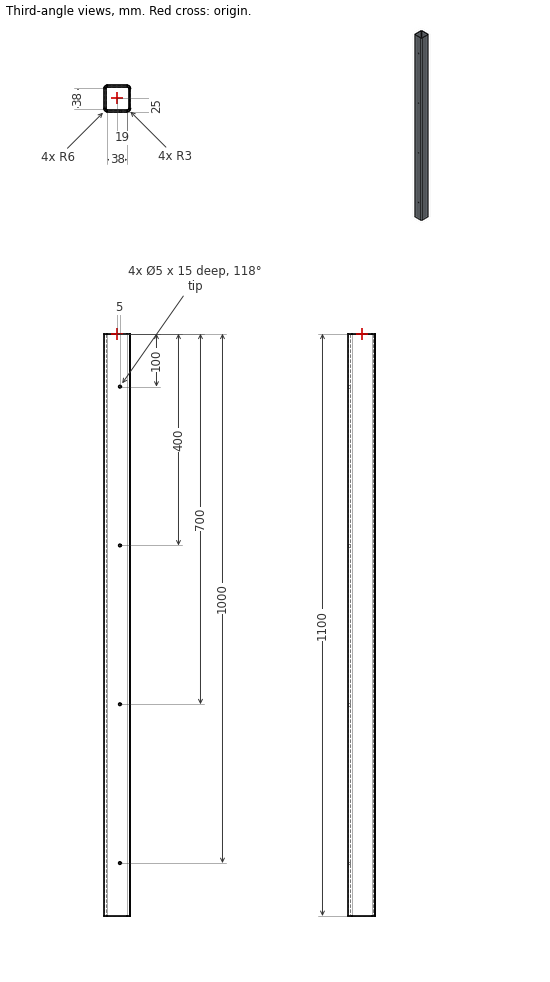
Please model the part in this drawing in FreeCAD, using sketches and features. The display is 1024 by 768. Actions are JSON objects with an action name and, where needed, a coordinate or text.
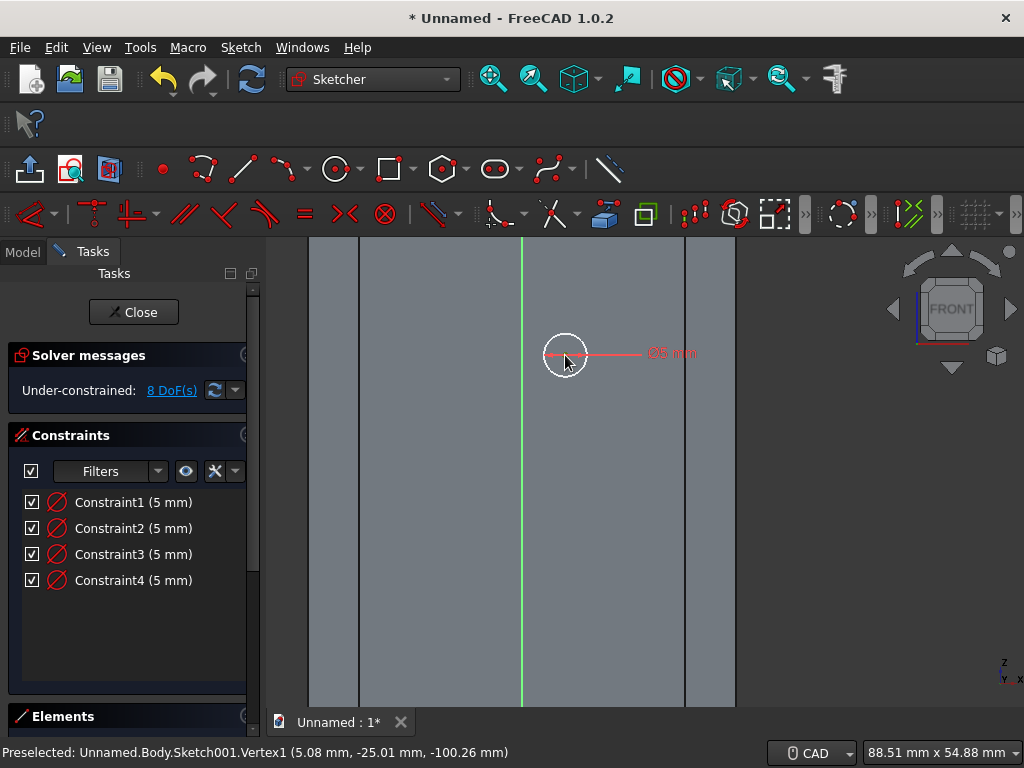
{"action": "left_click", "coordinate": [56, 214]}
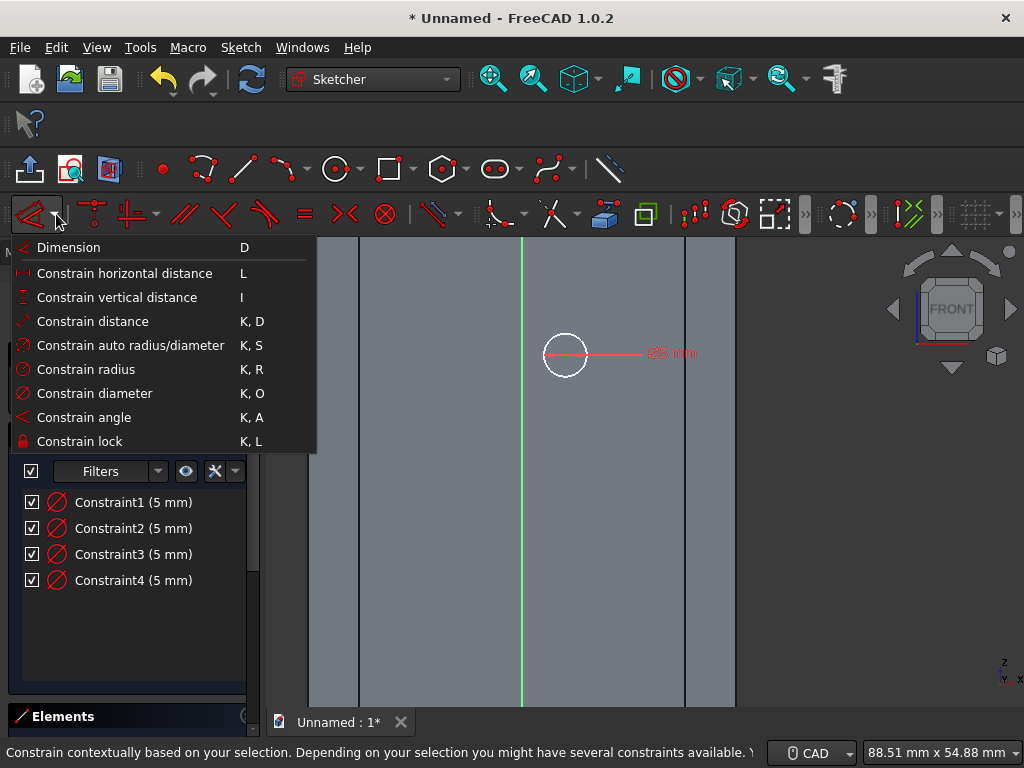
{"action": "left_click", "coordinate": [164, 273]}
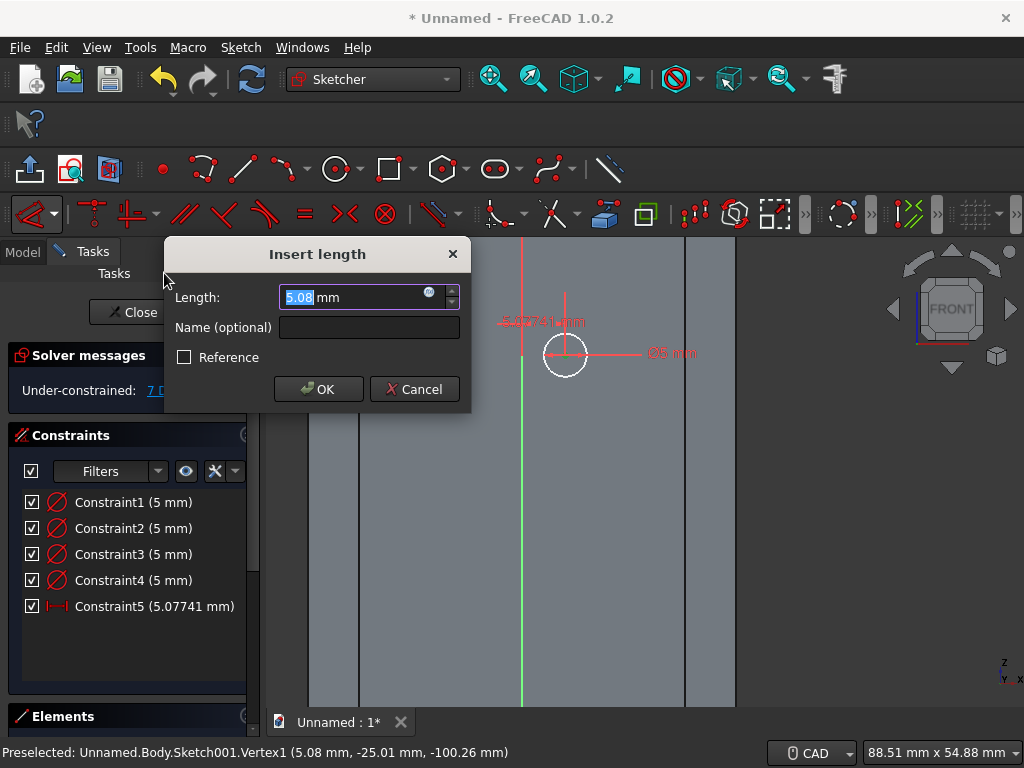
{"action": "type", "text": "5"}
{"action": "key", "text": "Return"}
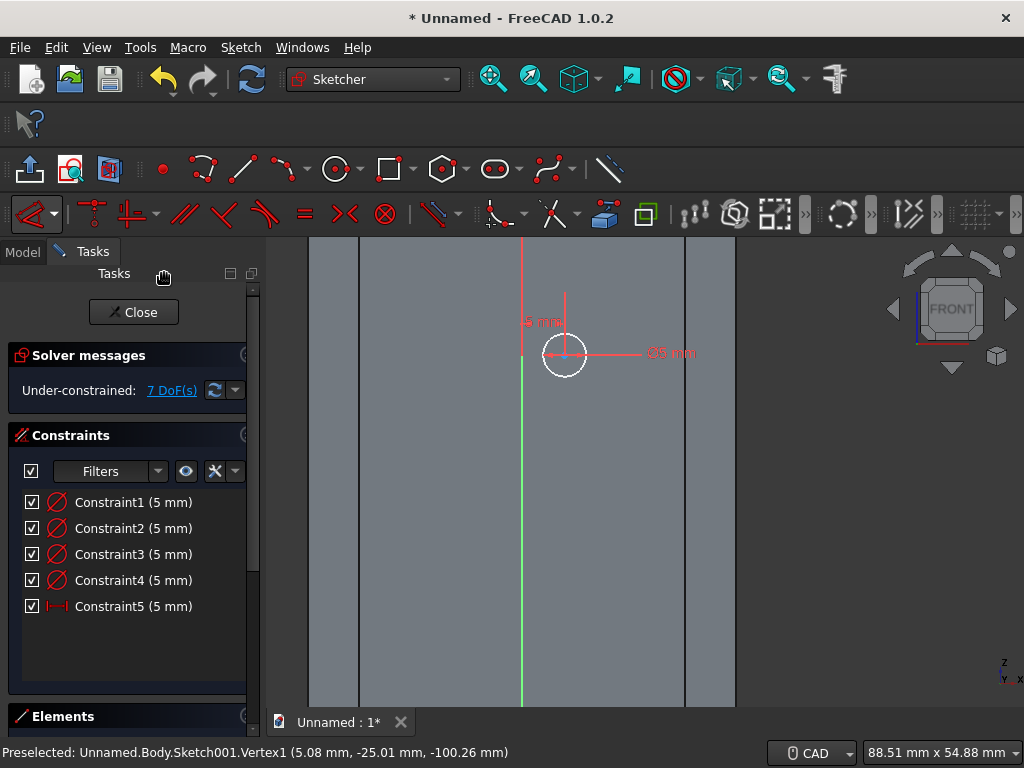
{"action": "scroll", "coordinate": [577, 331], "scroll_direction": "down", "scroll_amount": 16}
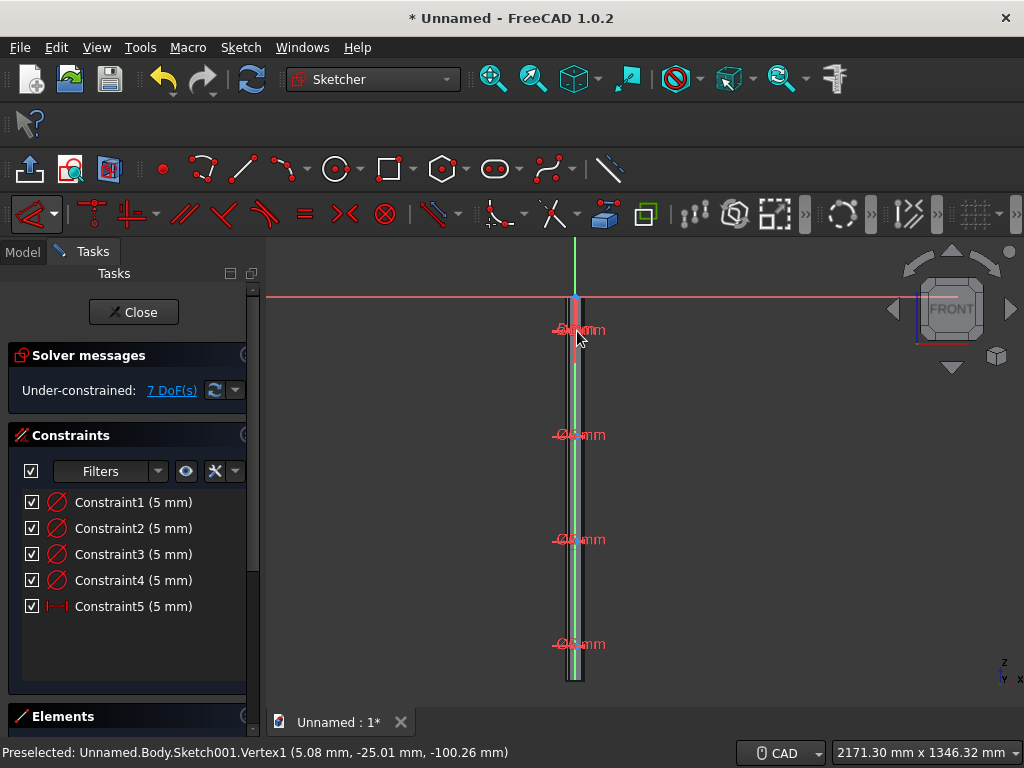
{"action": "scroll", "coordinate": [577, 437], "scroll_direction": "up", "scroll_amount": 16}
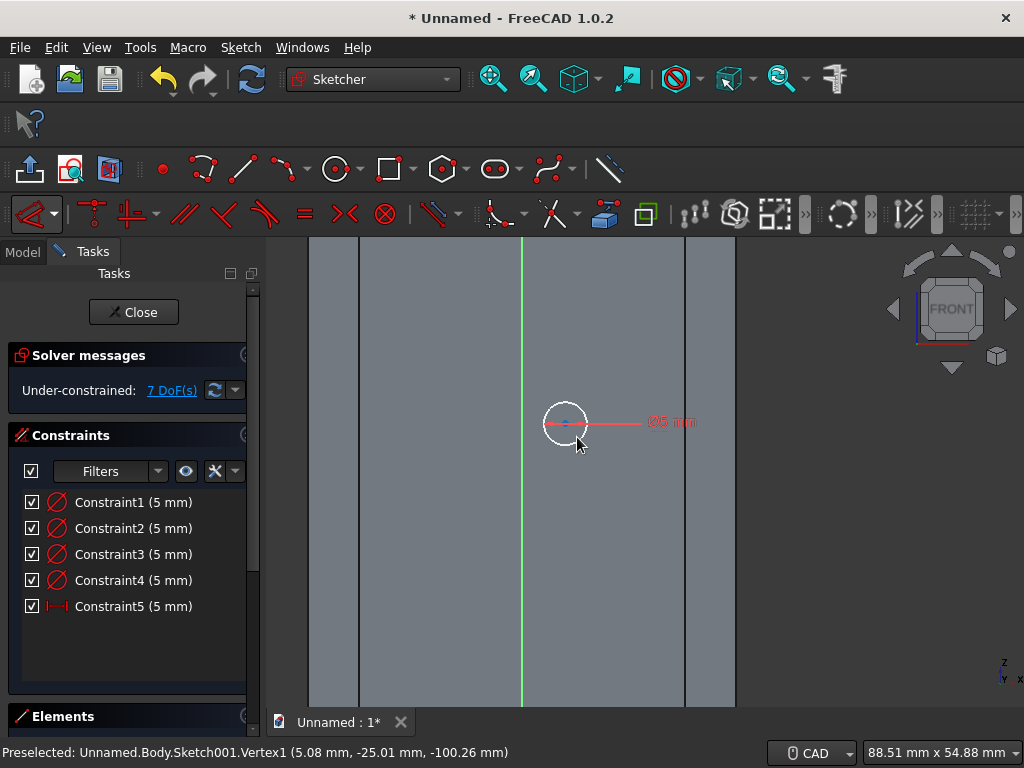
{"action": "left_click", "coordinate": [565, 424]}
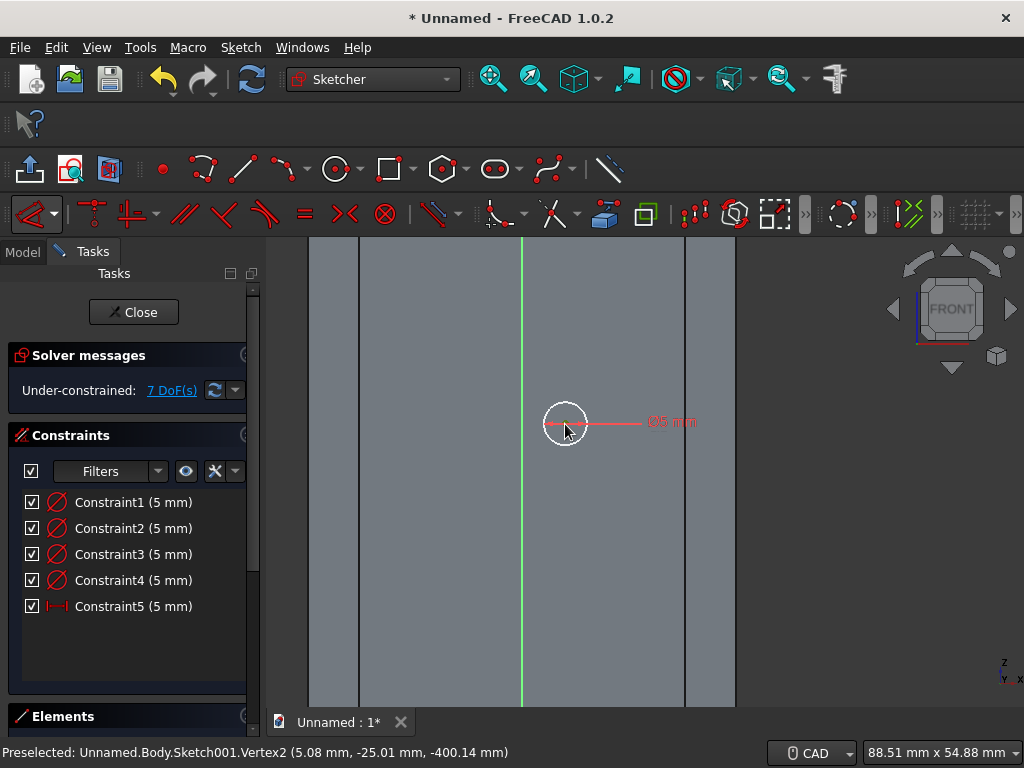
{"action": "key", "text": "l"}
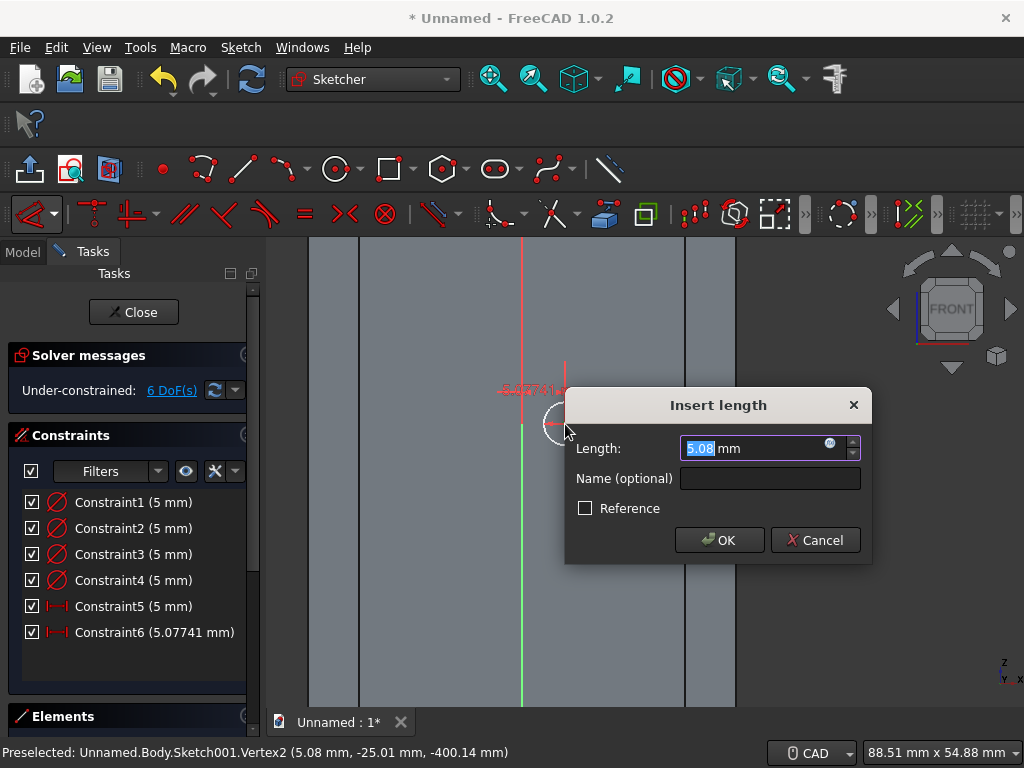
{"action": "type", "text": "5"}
{"action": "key", "text": "Return"}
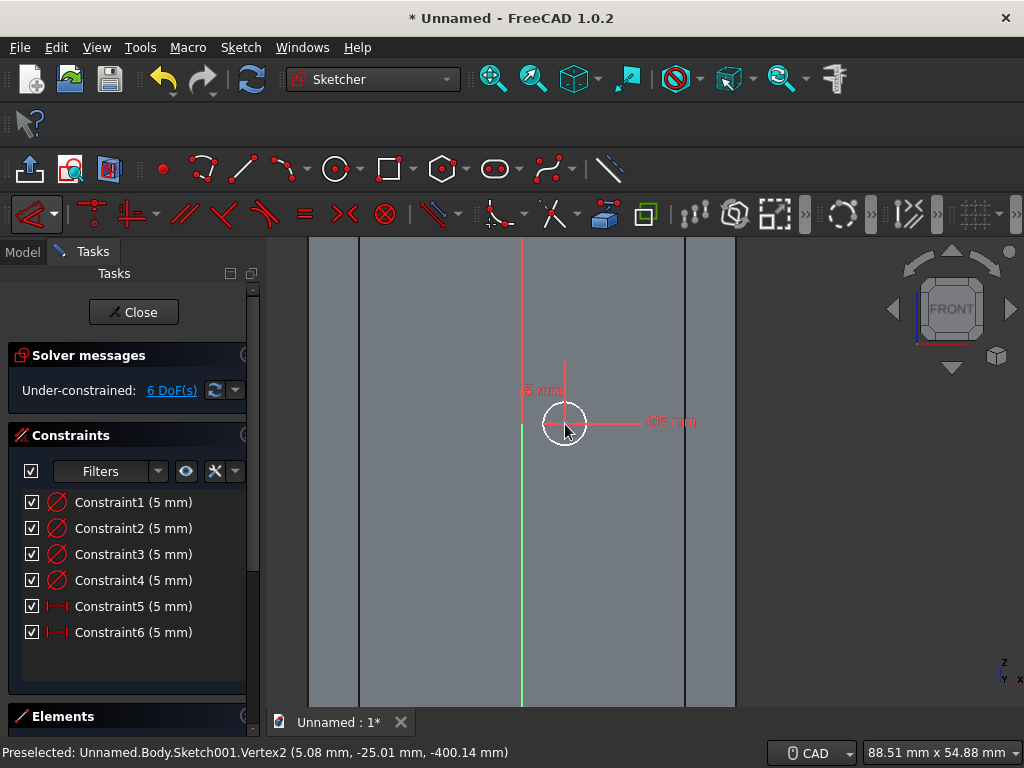
{"action": "scroll", "coordinate": [577, 437], "scroll_direction": "down", "scroll_amount": 16}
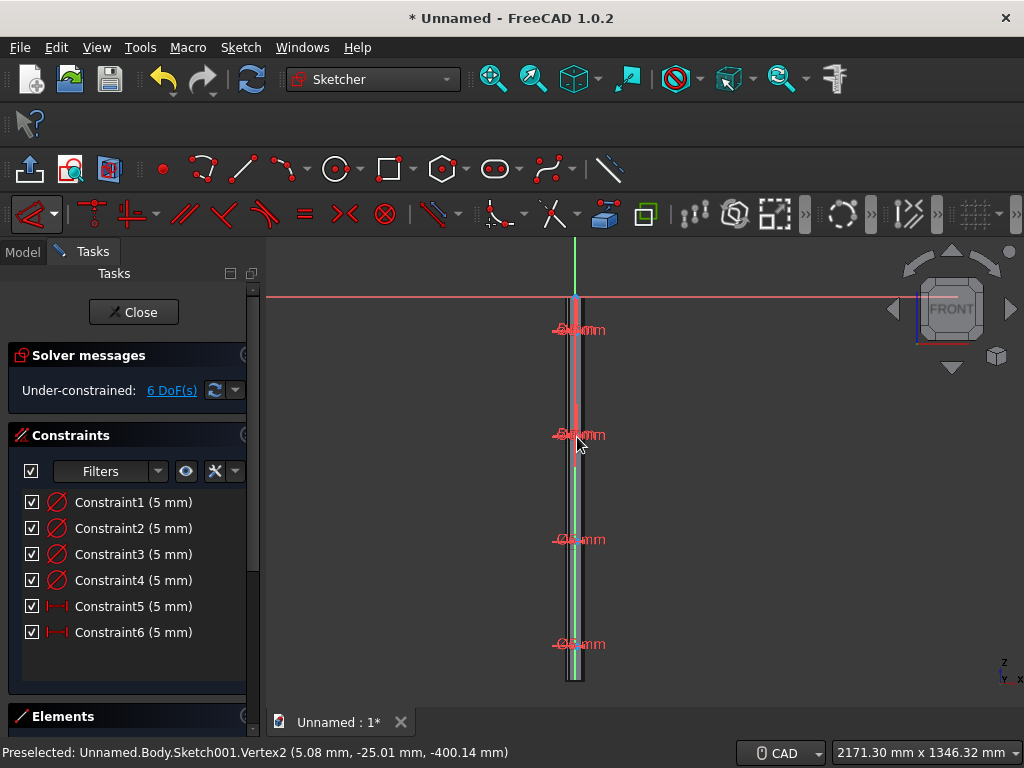
{"action": "scroll", "coordinate": [577, 542], "scroll_direction": "up", "scroll_amount": 16}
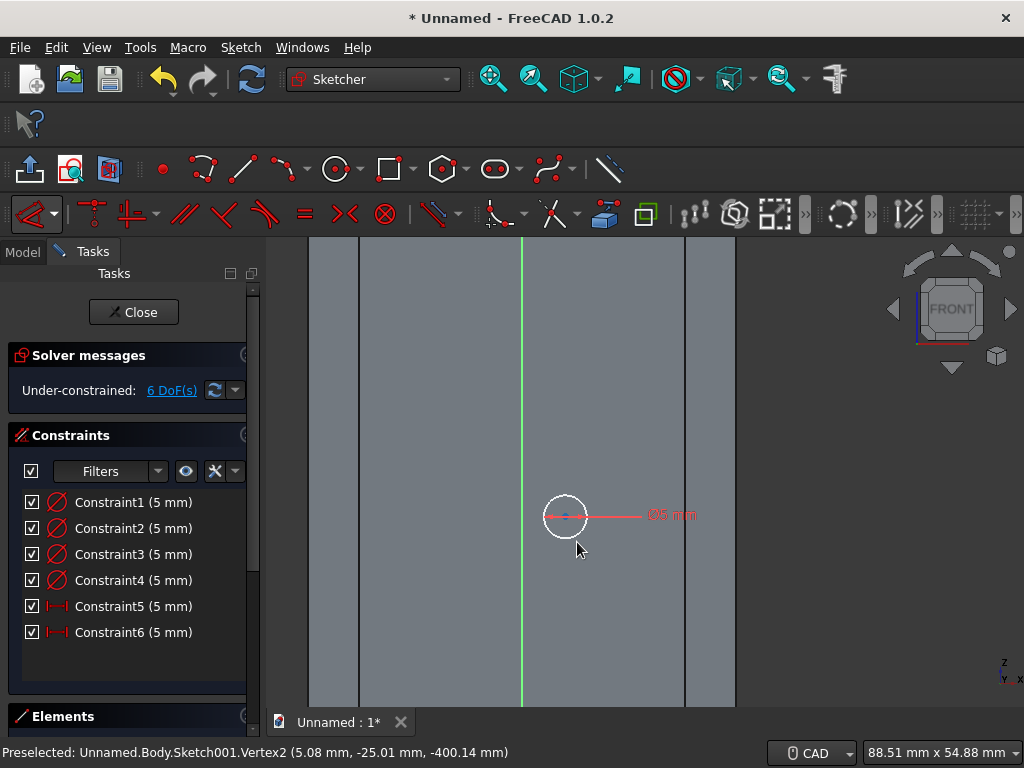
{"action": "left_click", "coordinate": [565, 517]}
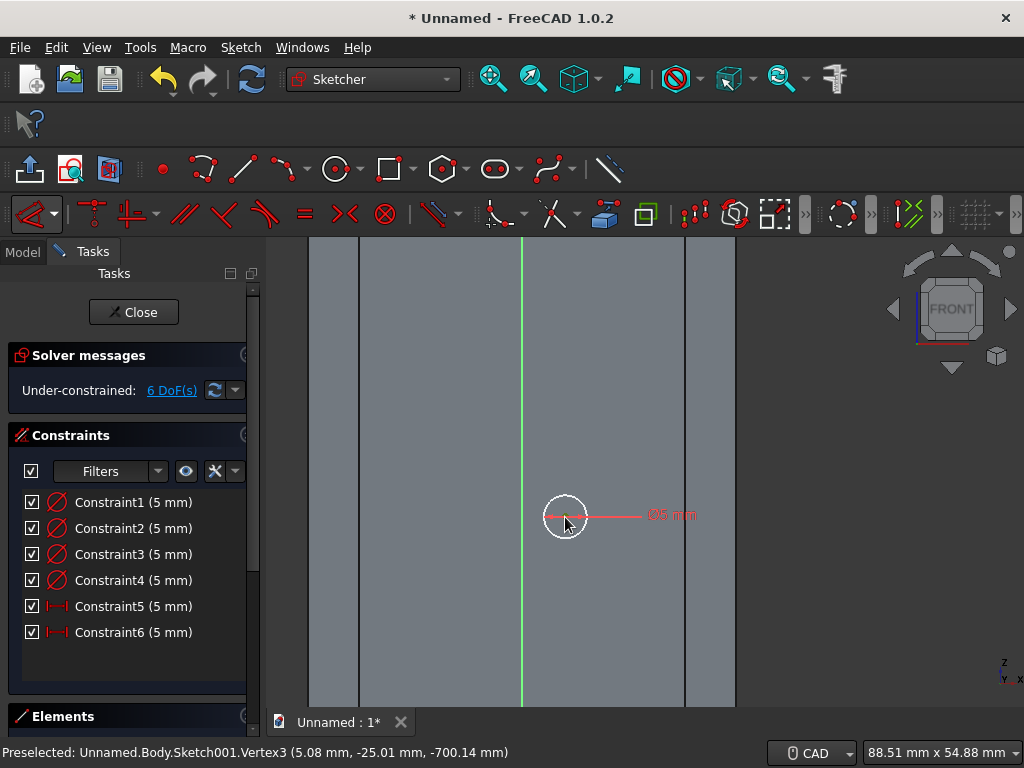
{"action": "key", "text": "l"}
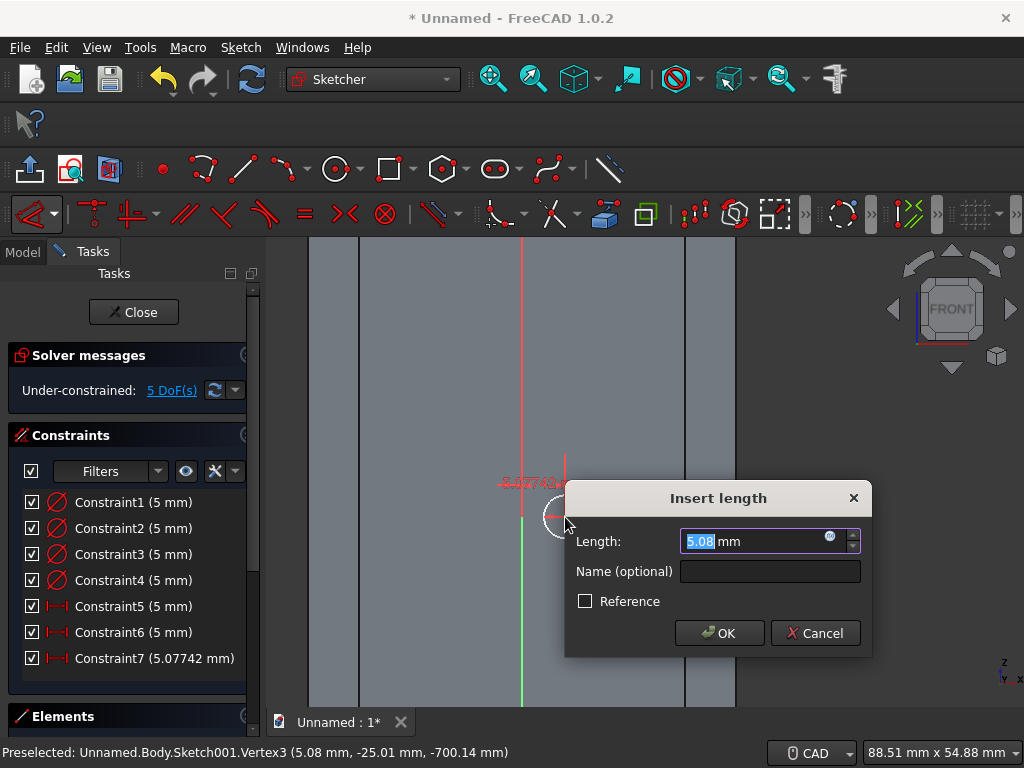
{"action": "type", "text": "5"}
{"action": "key", "text": "Return"}